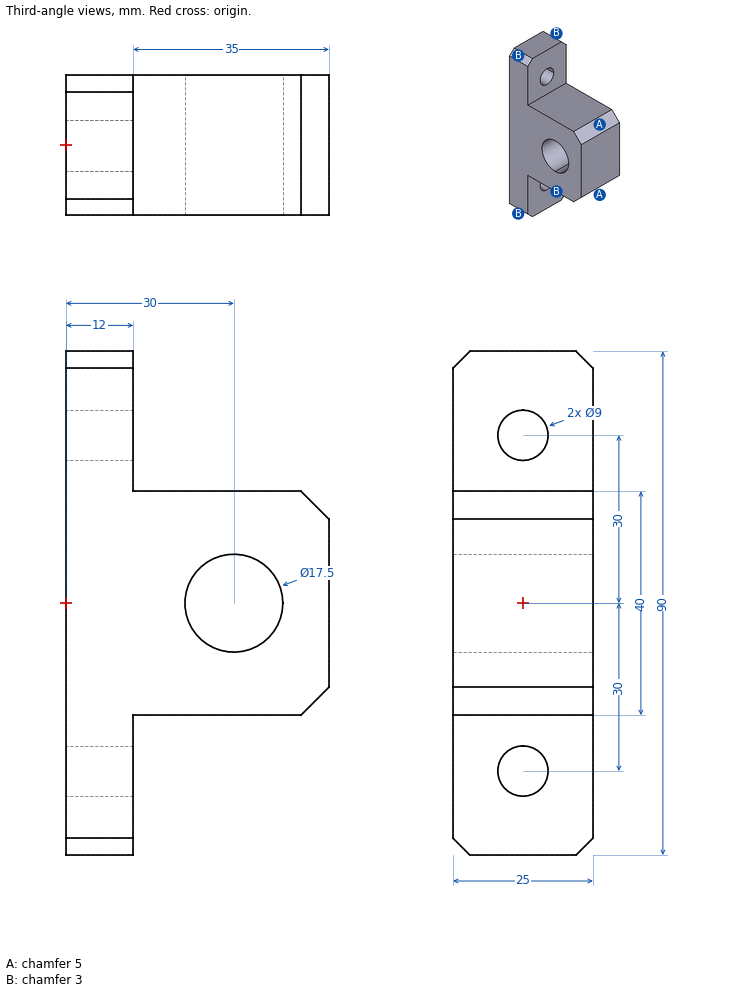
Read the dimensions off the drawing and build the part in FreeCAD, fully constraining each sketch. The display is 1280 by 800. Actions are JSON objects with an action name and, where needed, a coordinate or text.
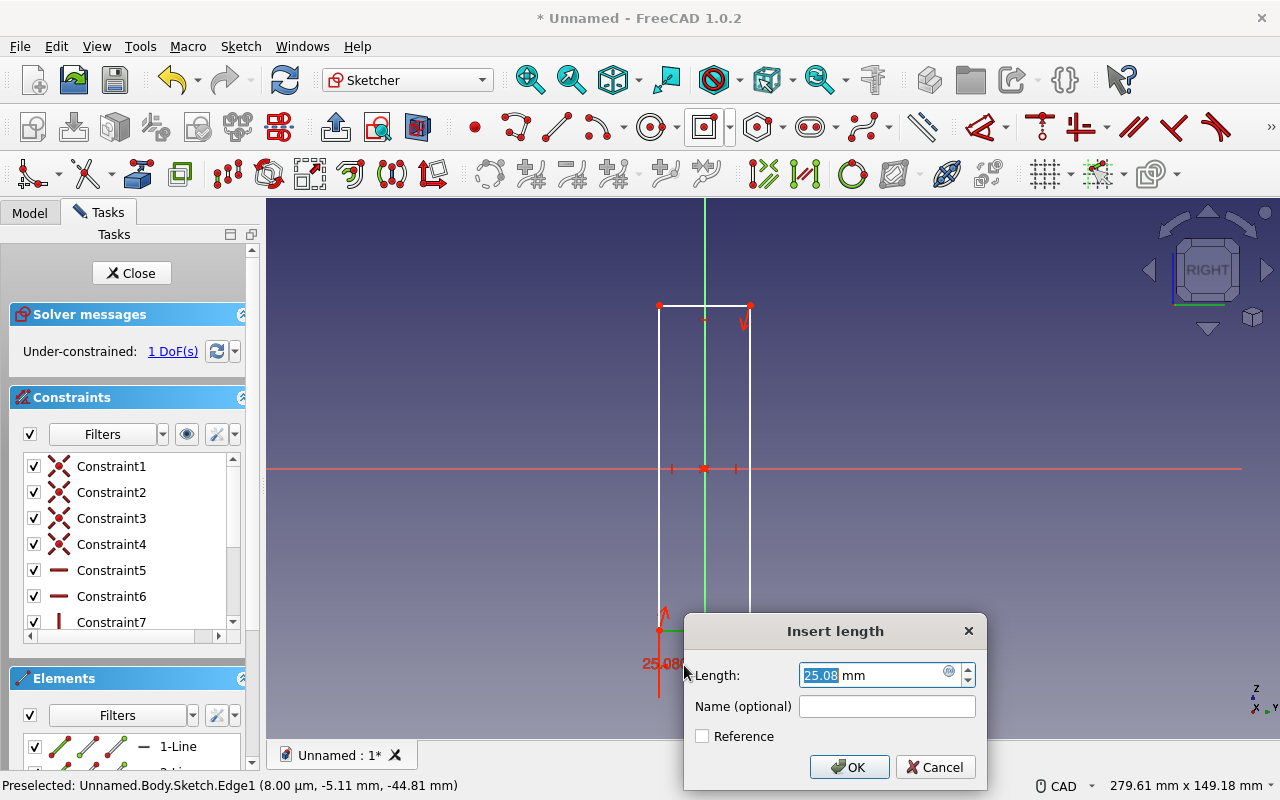
{"action": "type", "text": "25"}
{"action": "key", "text": "Return"}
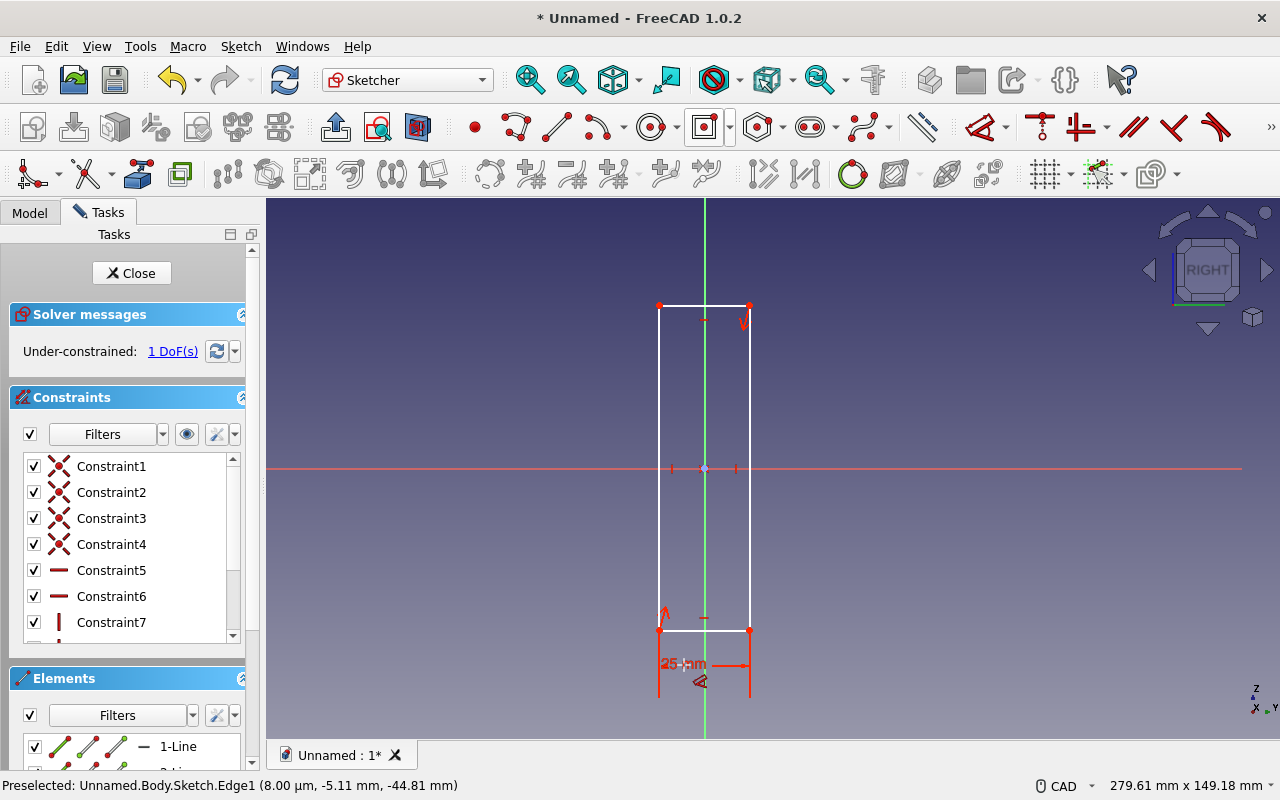
{"action": "left_click", "coordinate": [750, 534]}
{"action": "left_click", "coordinate": [784, 394]}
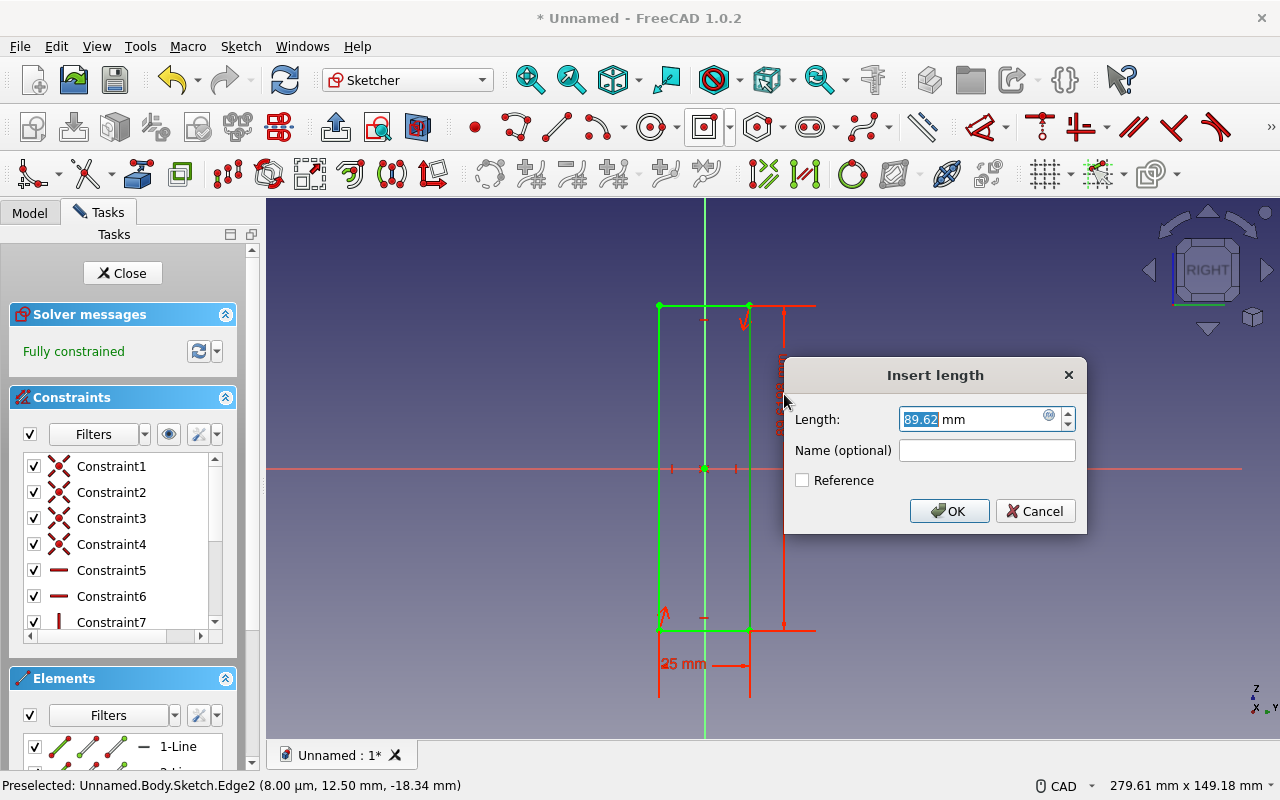
{"action": "type", "text": "90"}
{"action": "key", "text": "Return"}
{"action": "key", "text": "Escape"}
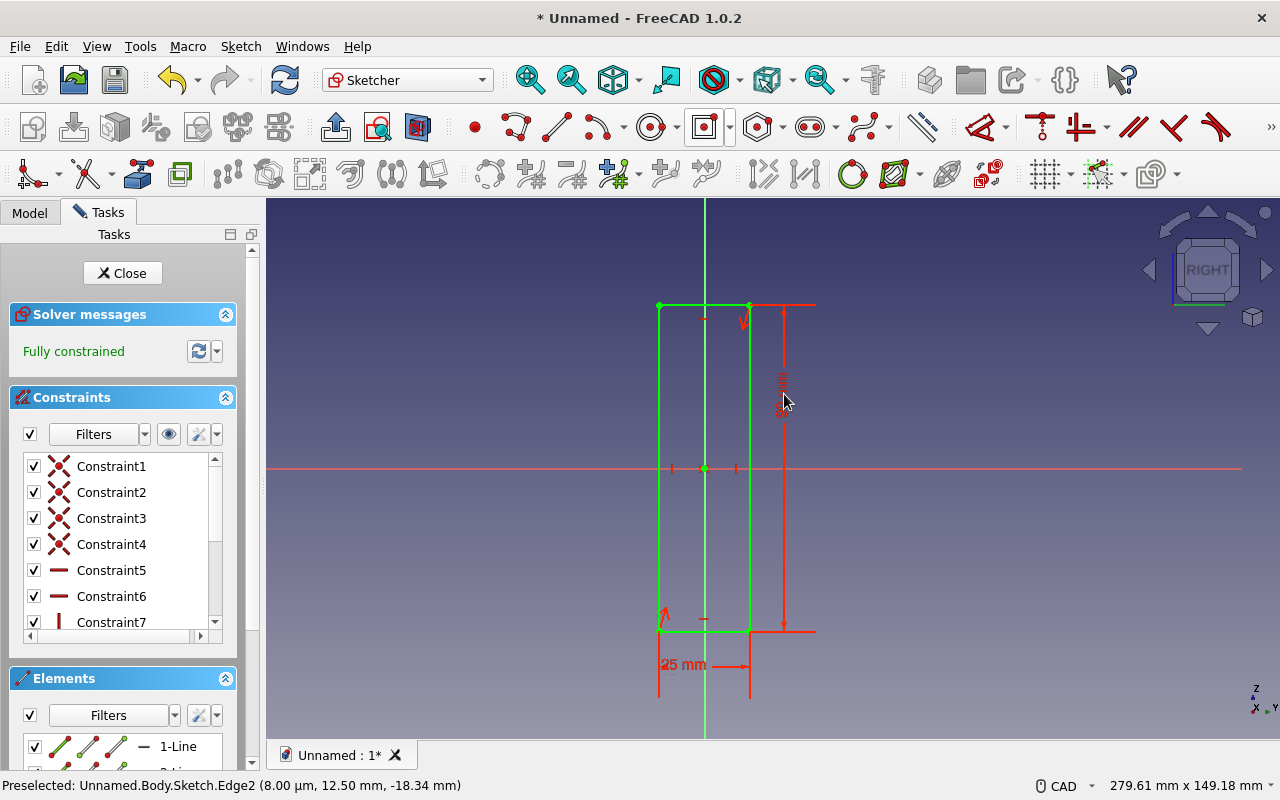
{"action": "left_click", "coordinate": [123, 273]}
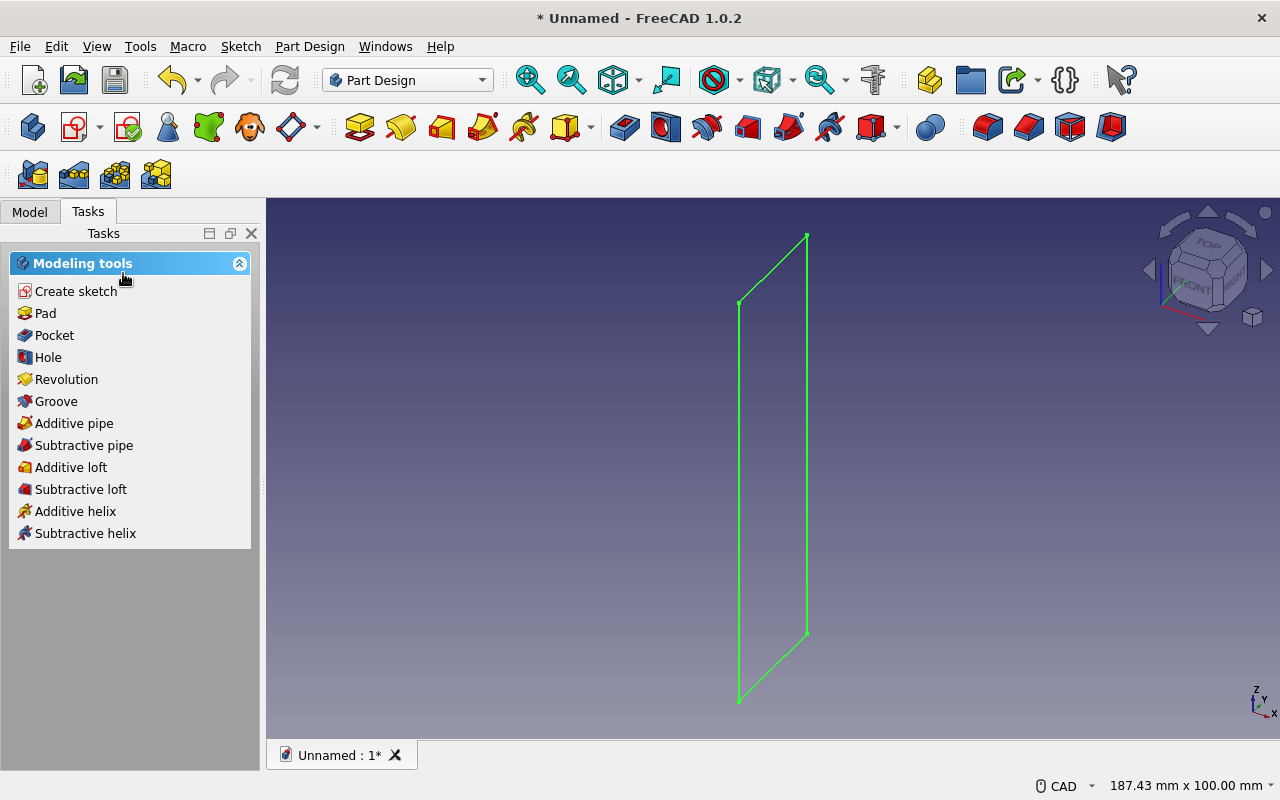
{"action": "left_click", "coordinate": [360, 128]}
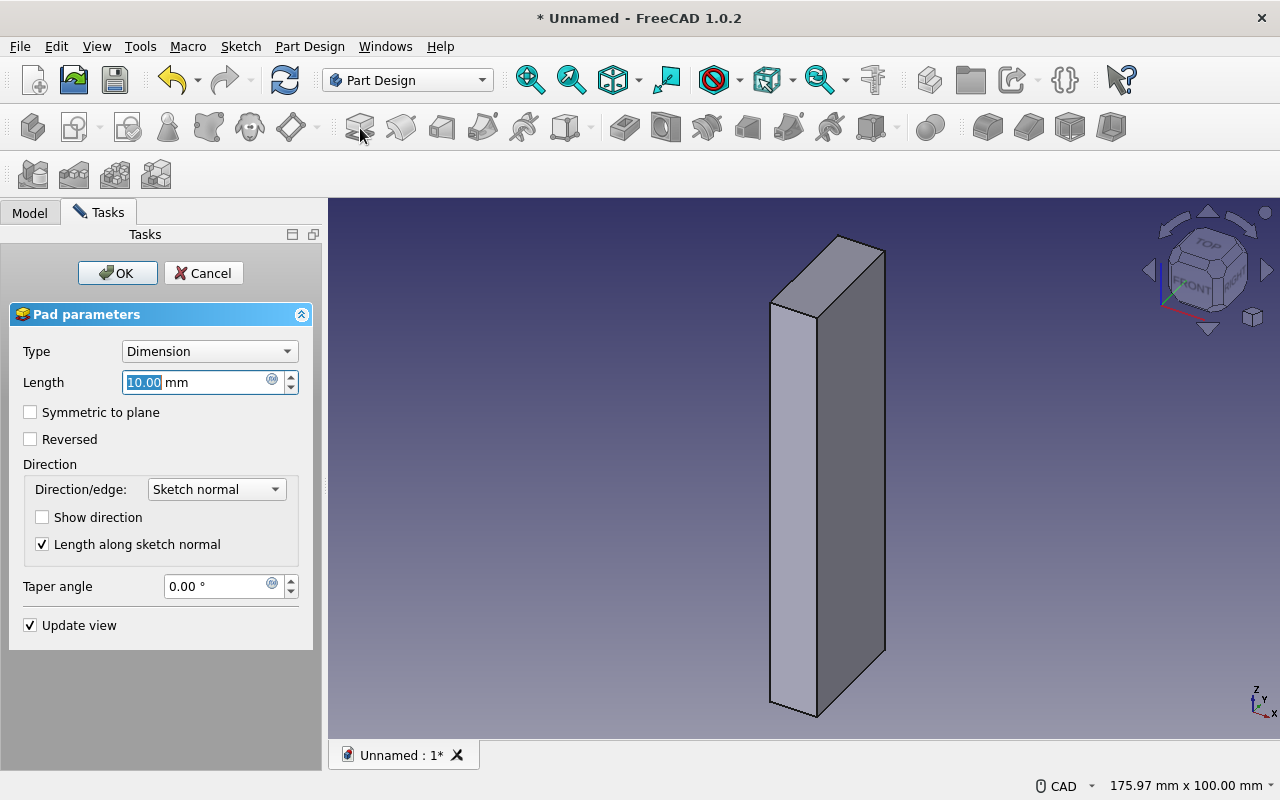
{"action": "type", "text": "12"}
{"action": "key", "text": "Tab"}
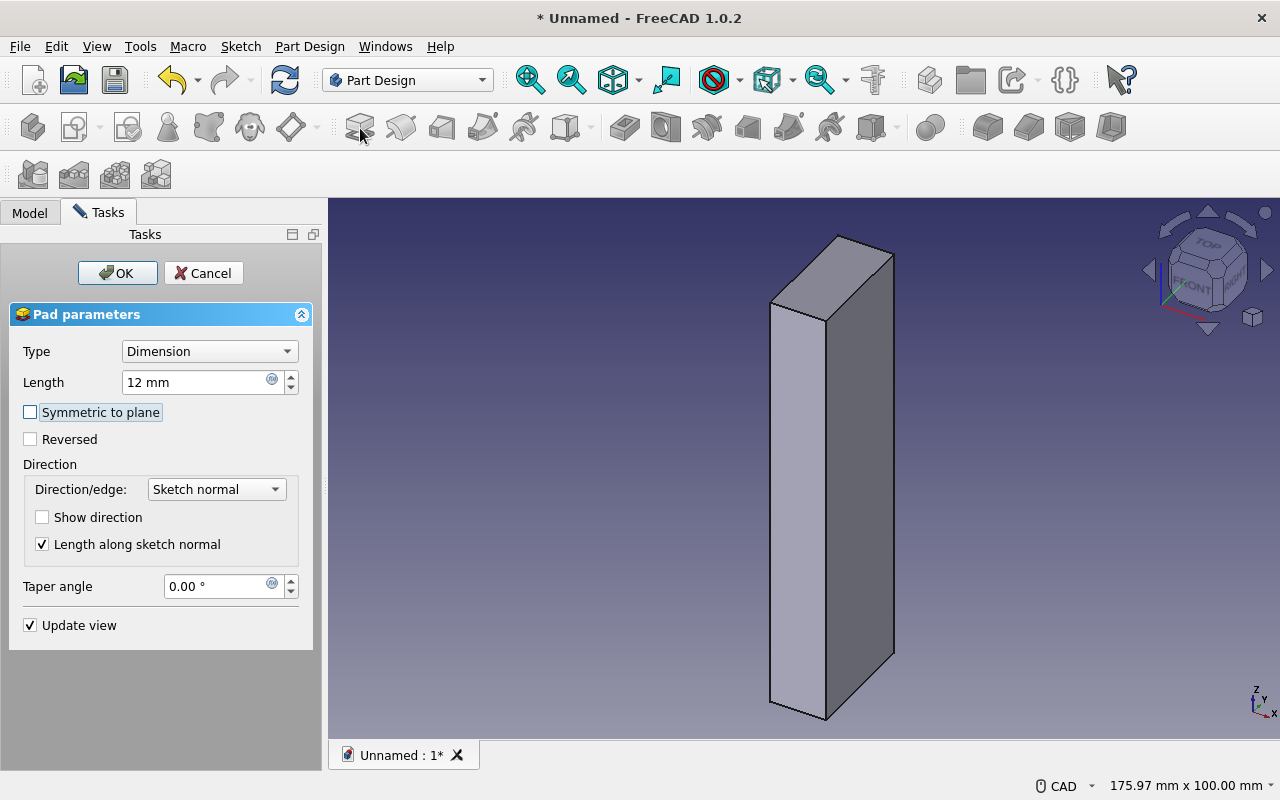
{"action": "left_click", "coordinate": [118, 273]}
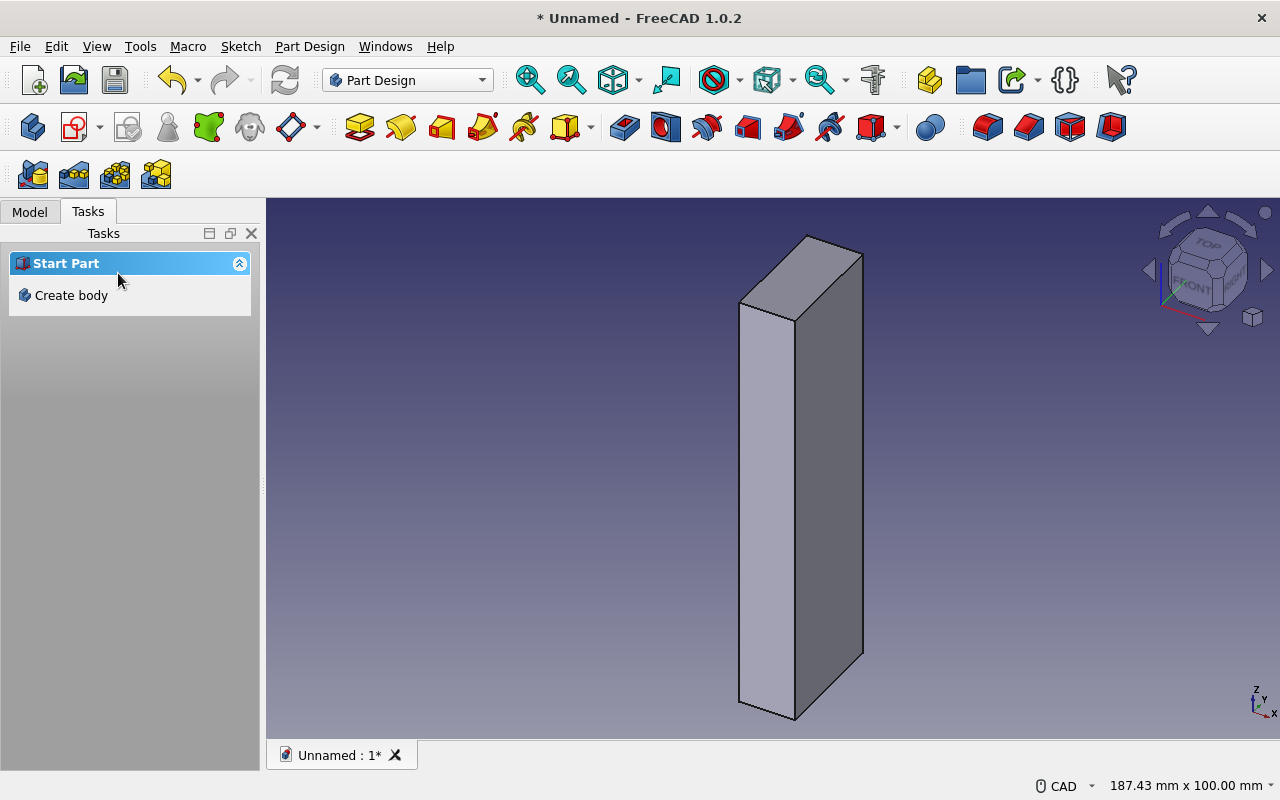
{"action": "left_click", "coordinate": [829, 543]}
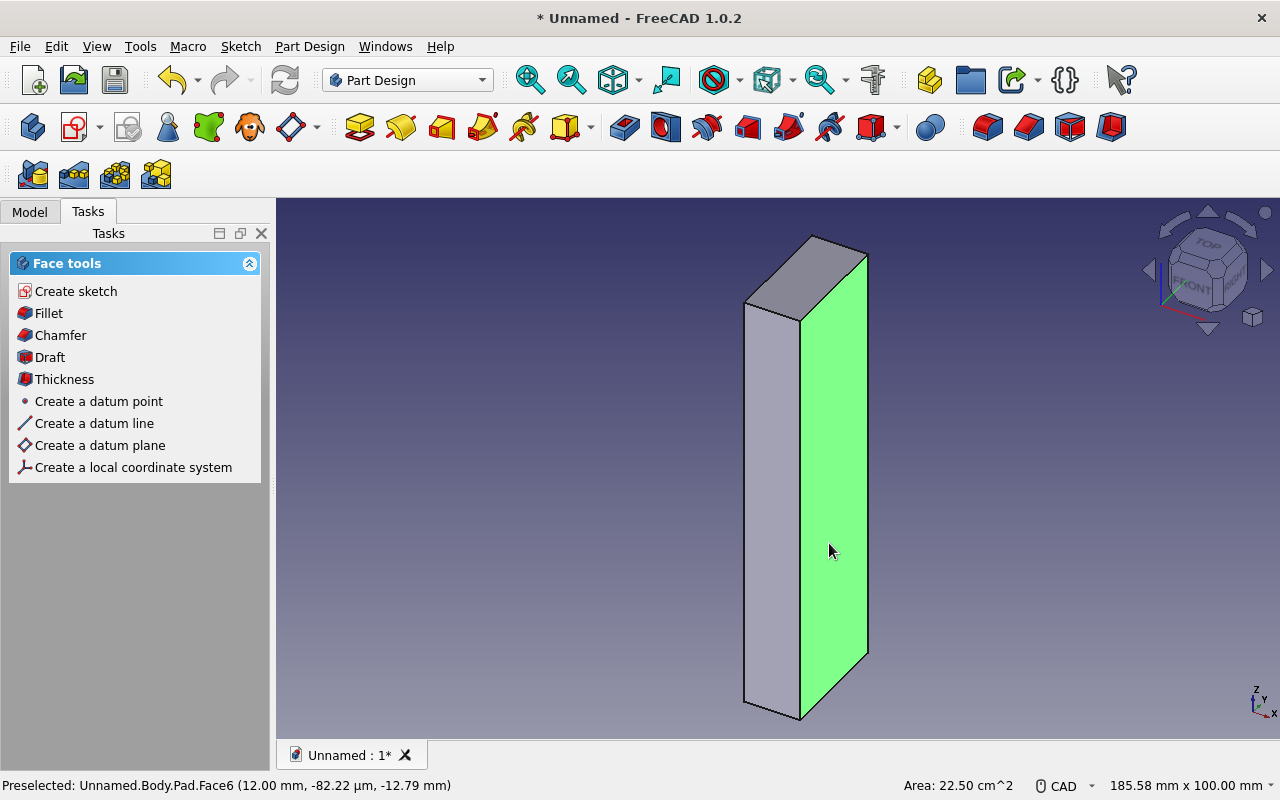
{"action": "left_click", "coordinate": [74, 128]}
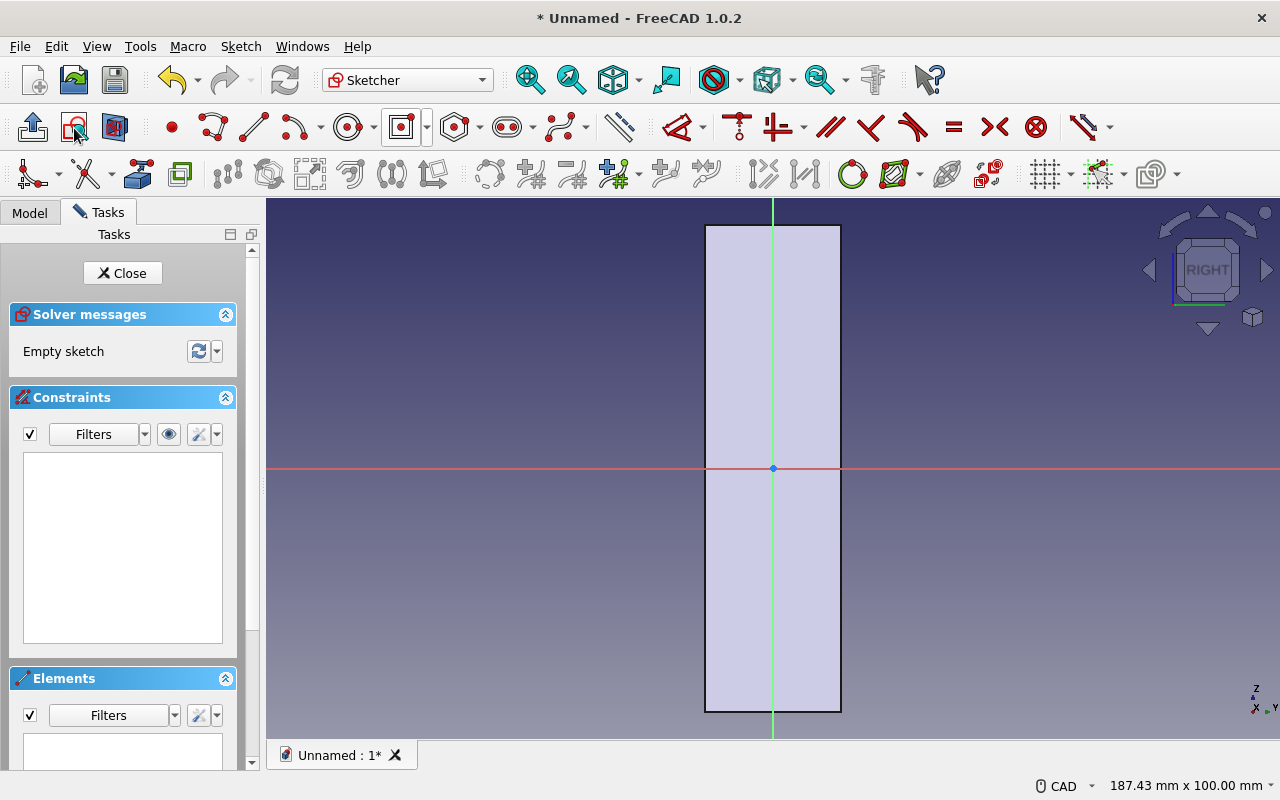
{"action": "scroll", "coordinate": [912, 469], "scroll_direction": "up", "scroll_amount": 2}